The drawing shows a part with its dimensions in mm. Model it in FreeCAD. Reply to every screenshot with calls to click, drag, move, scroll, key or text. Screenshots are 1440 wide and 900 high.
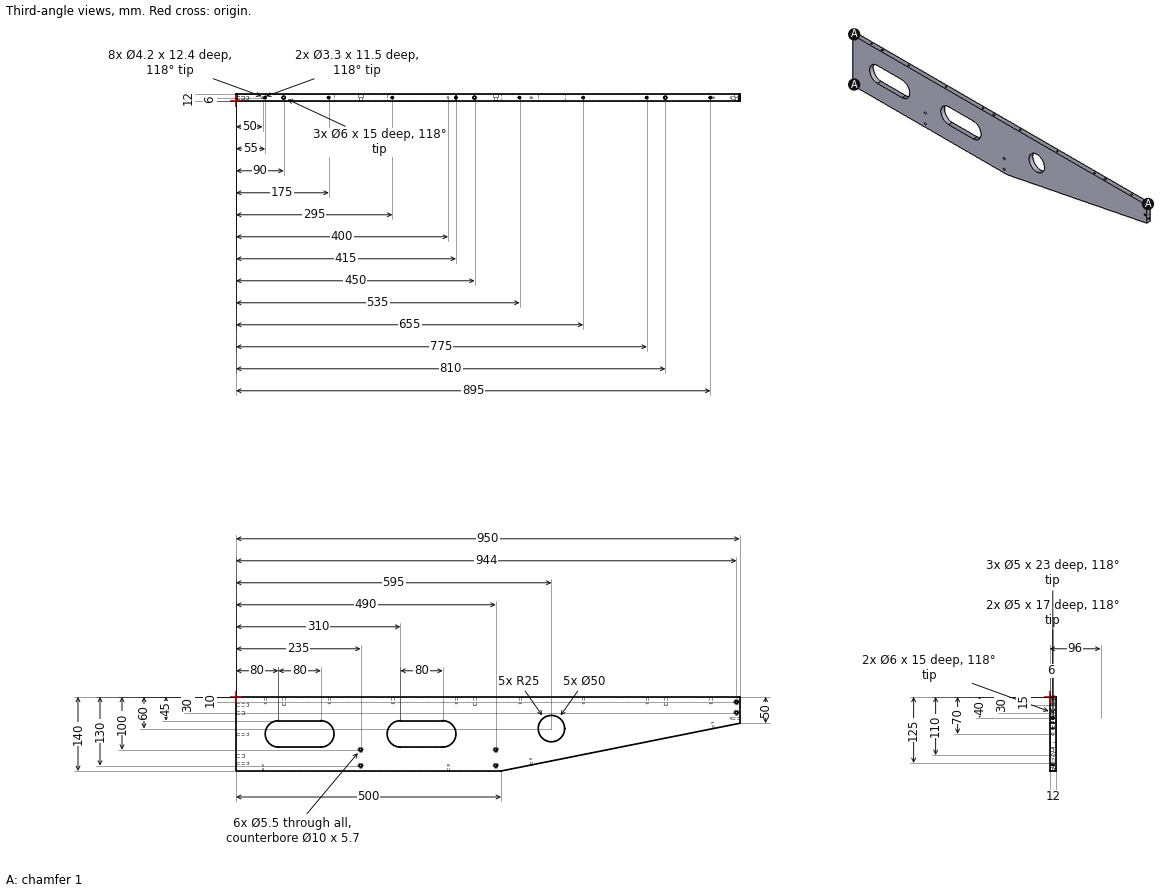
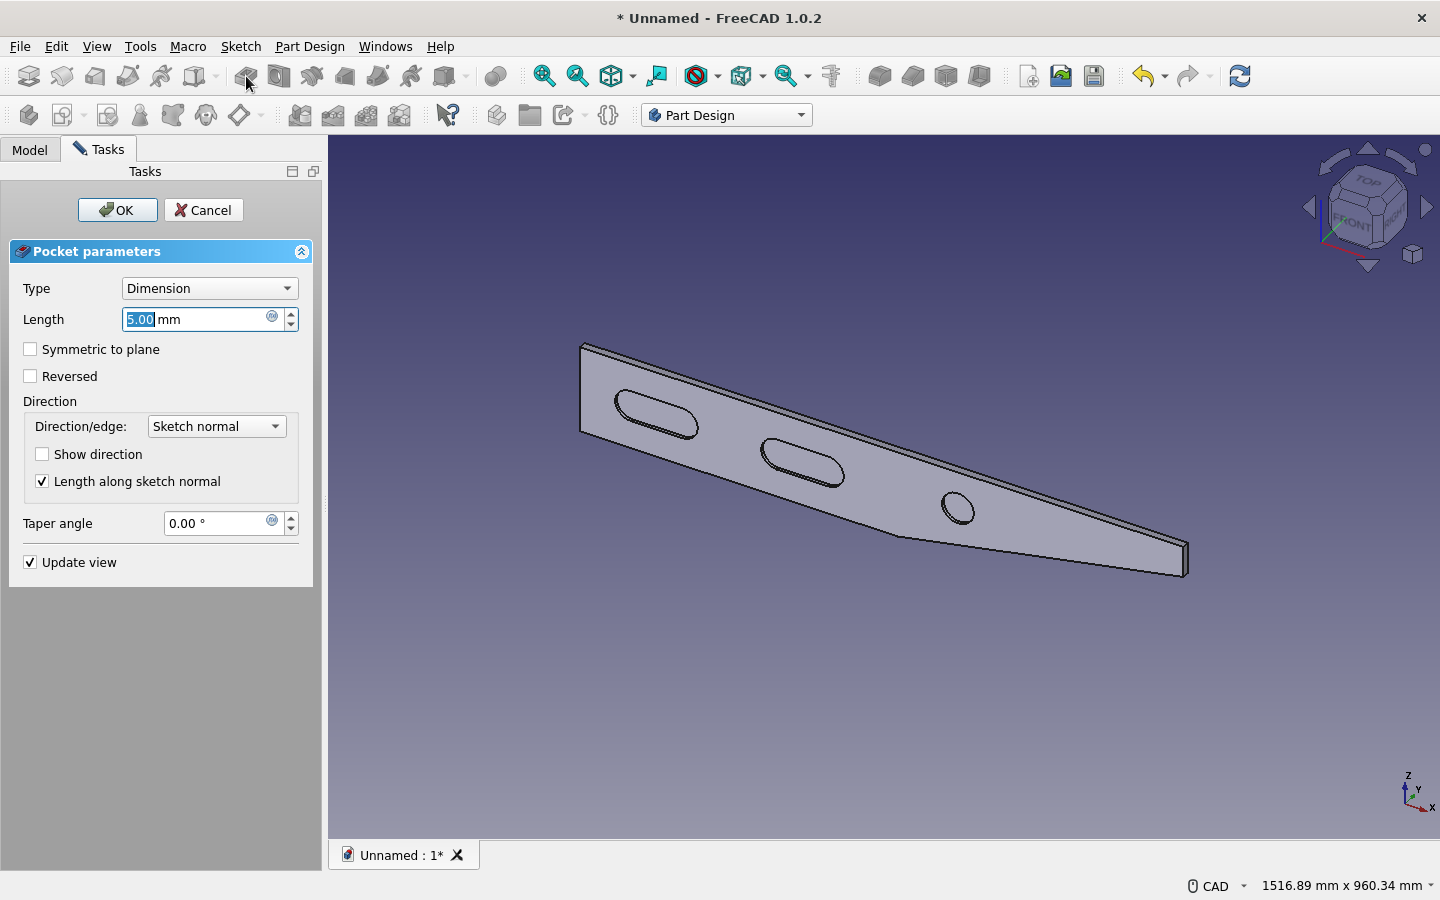
text(12)
key(Tab)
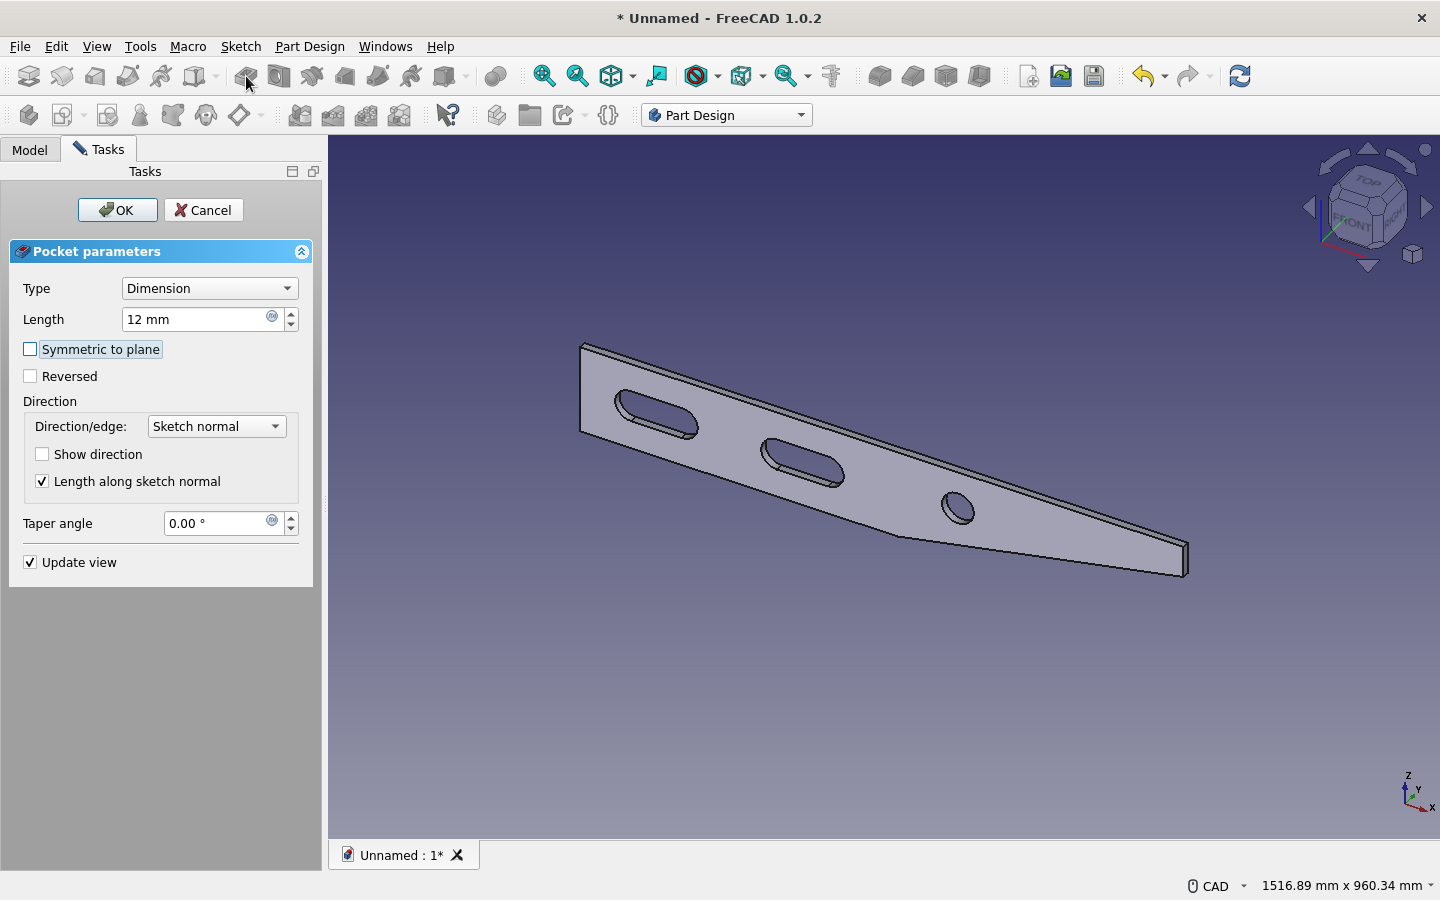
click(118, 210)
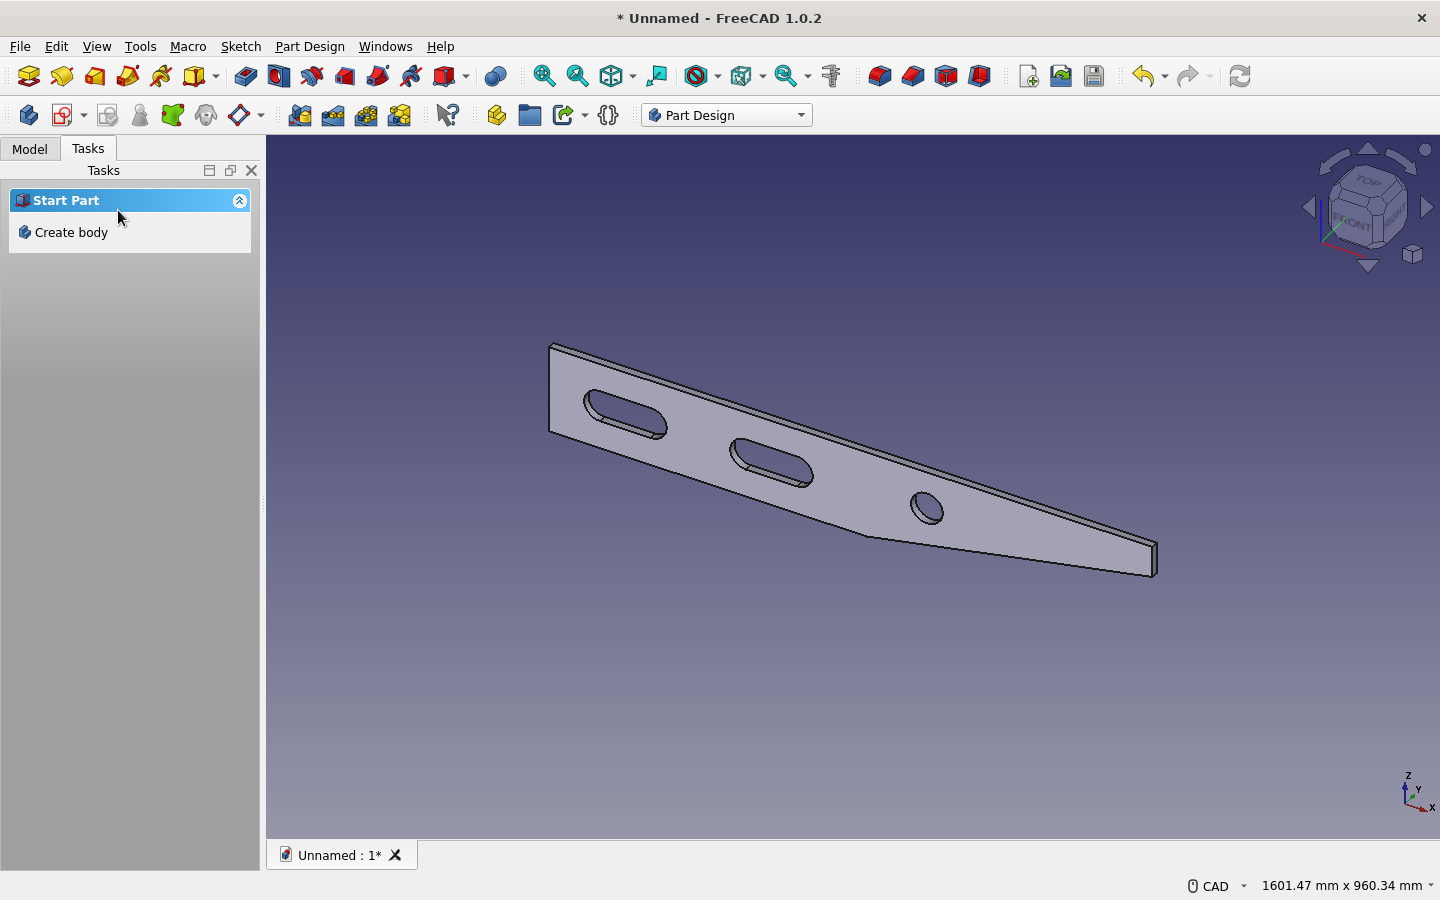
key(5)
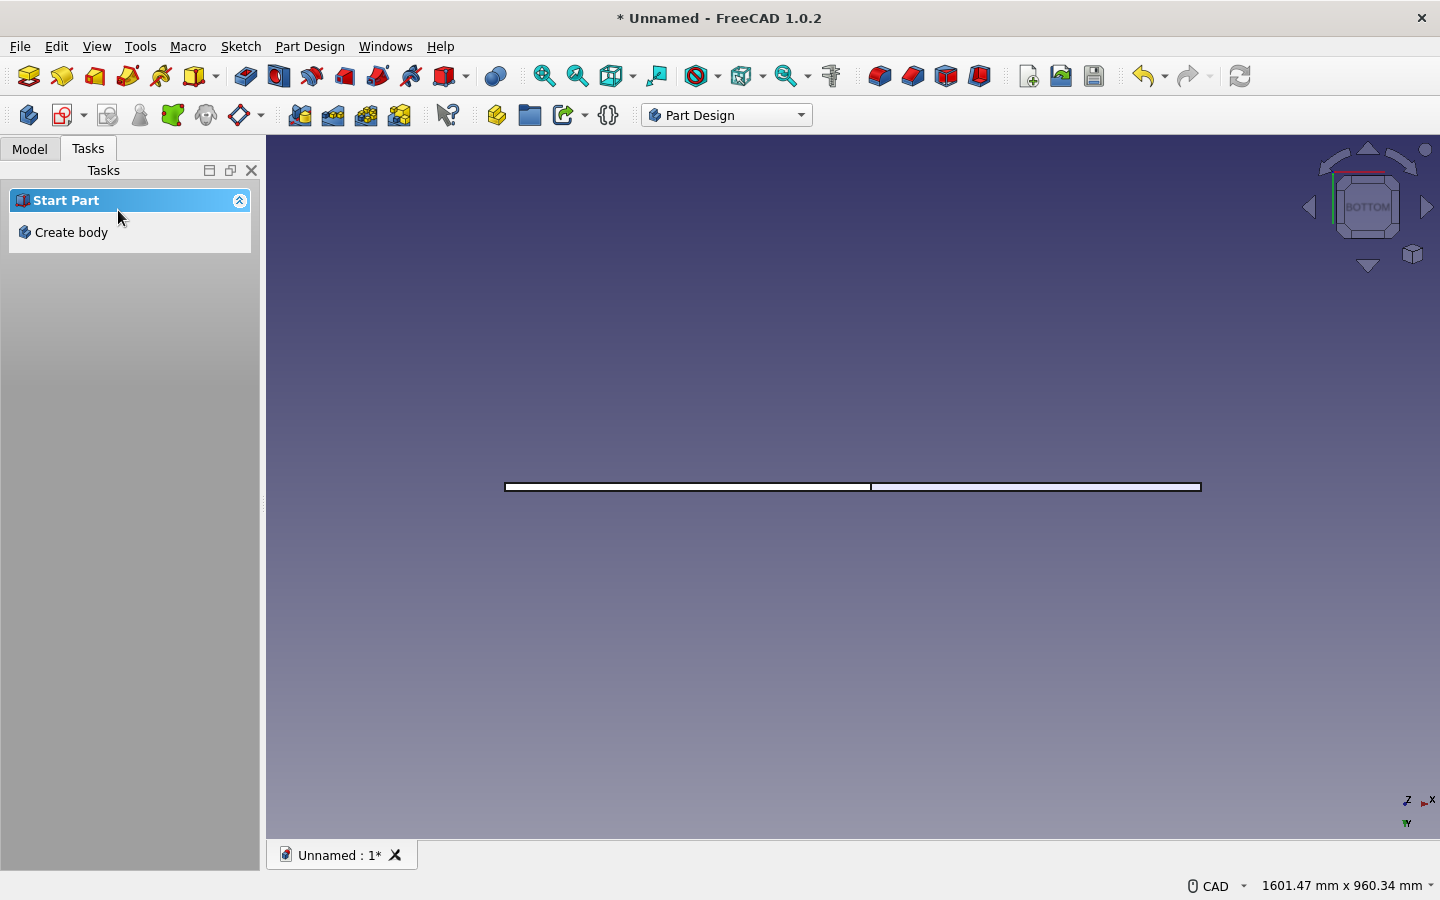
scroll(845, 486, up, 6)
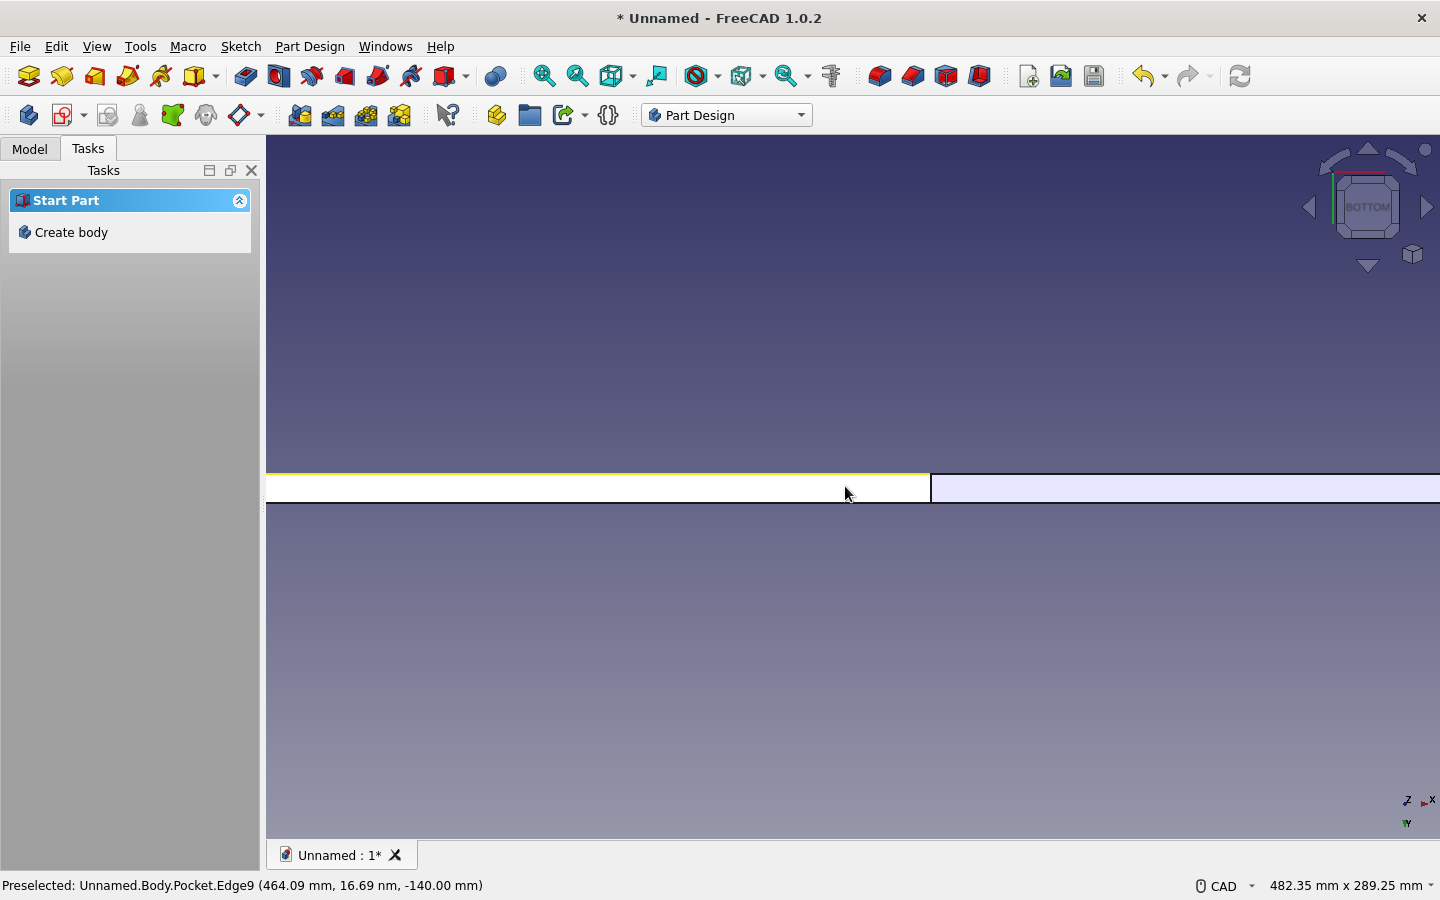
click(844, 487)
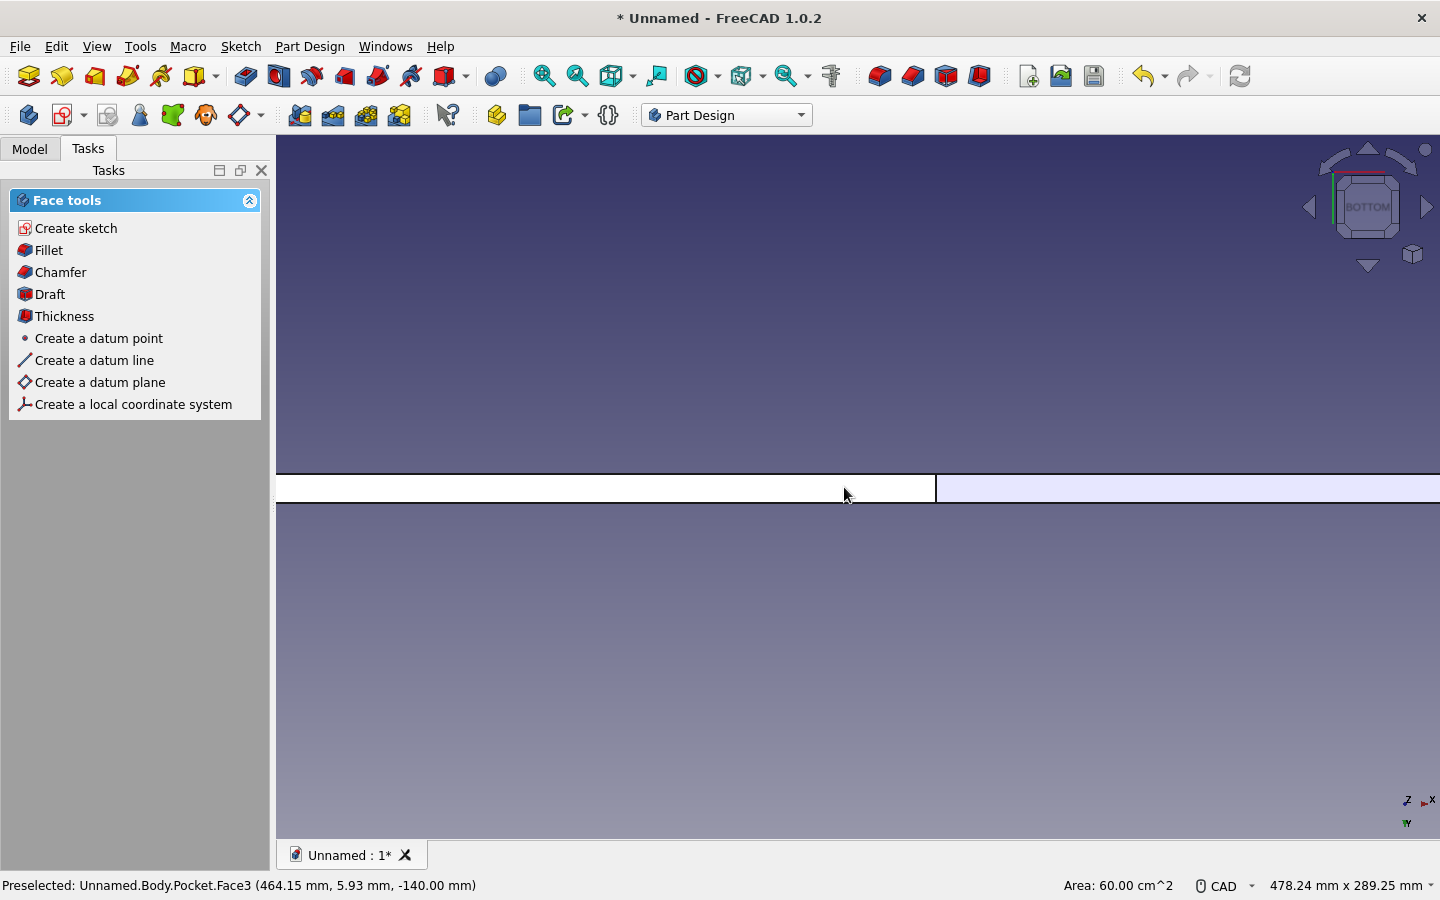
click(62, 116)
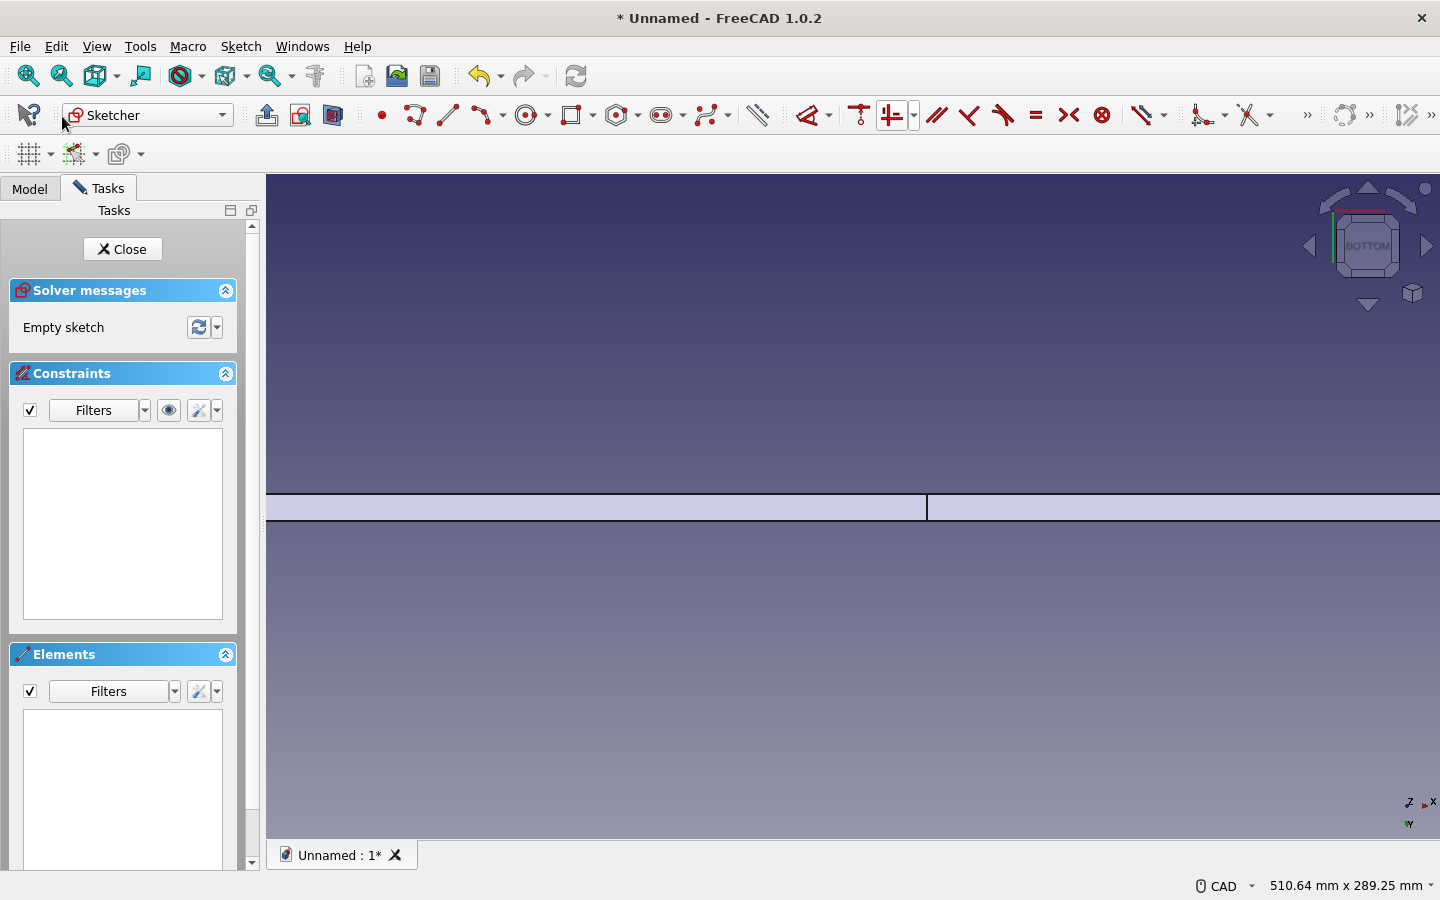
scroll(1275, 511, down, 3)